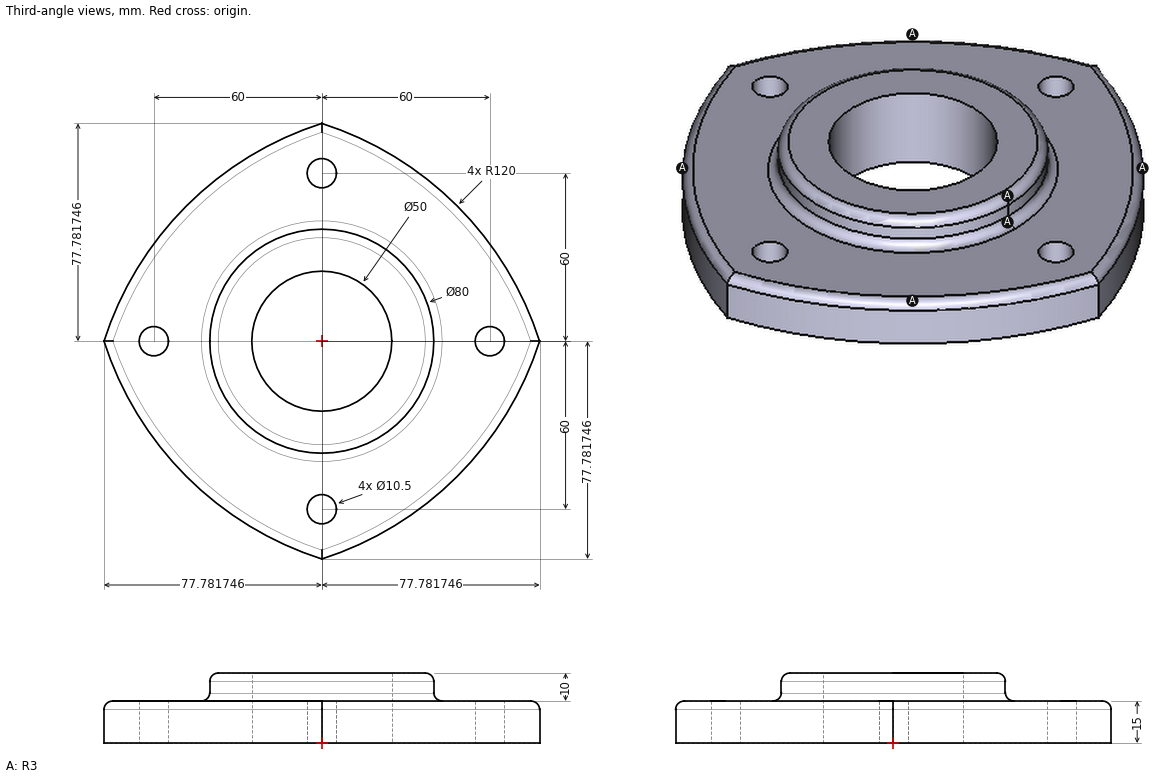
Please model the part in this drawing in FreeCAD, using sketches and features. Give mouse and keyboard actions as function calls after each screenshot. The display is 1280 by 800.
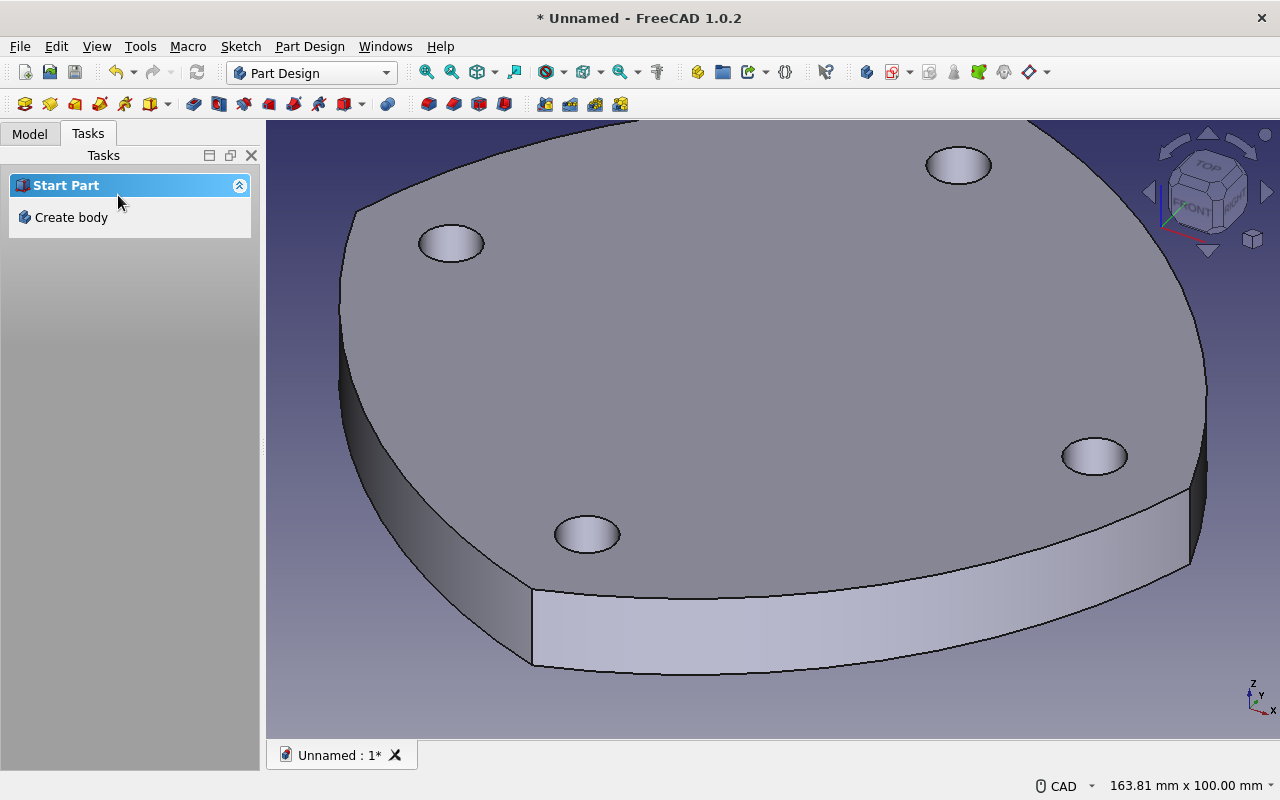
key(v)
key(f)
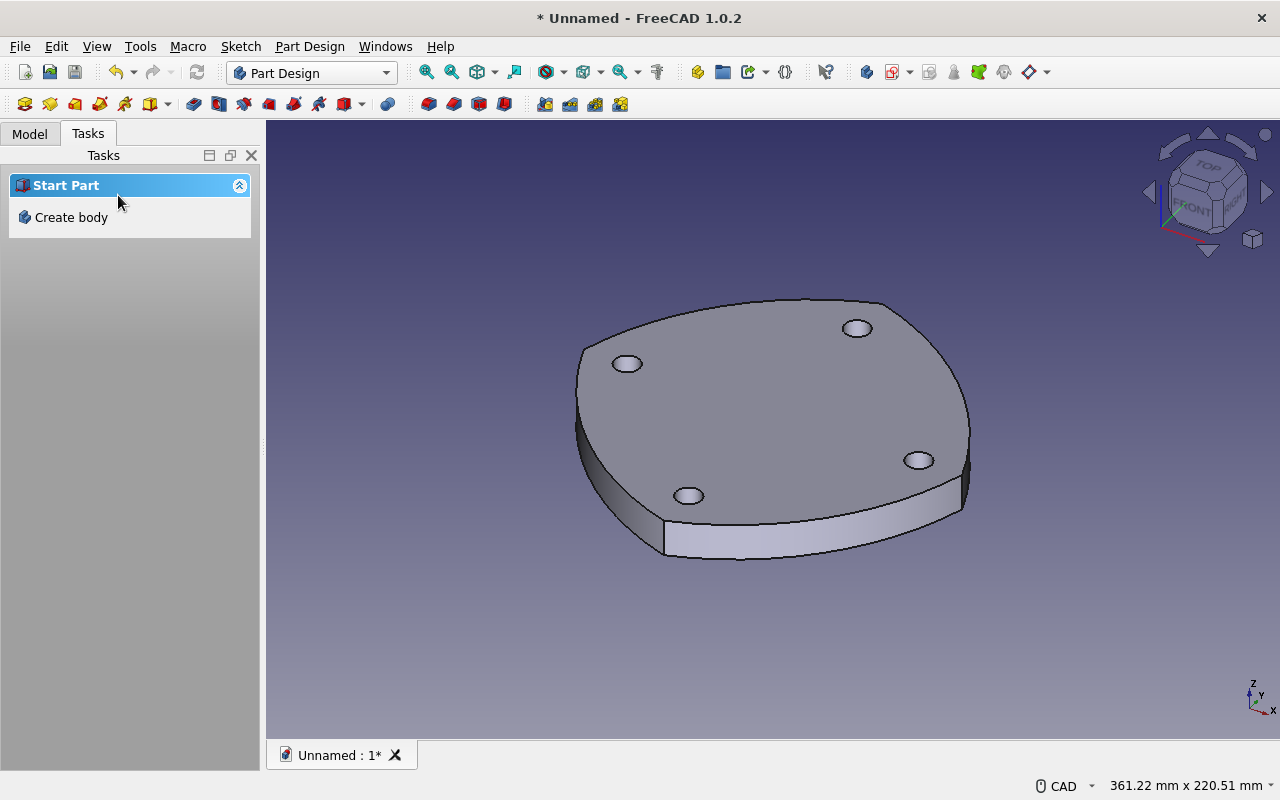
click(773, 411)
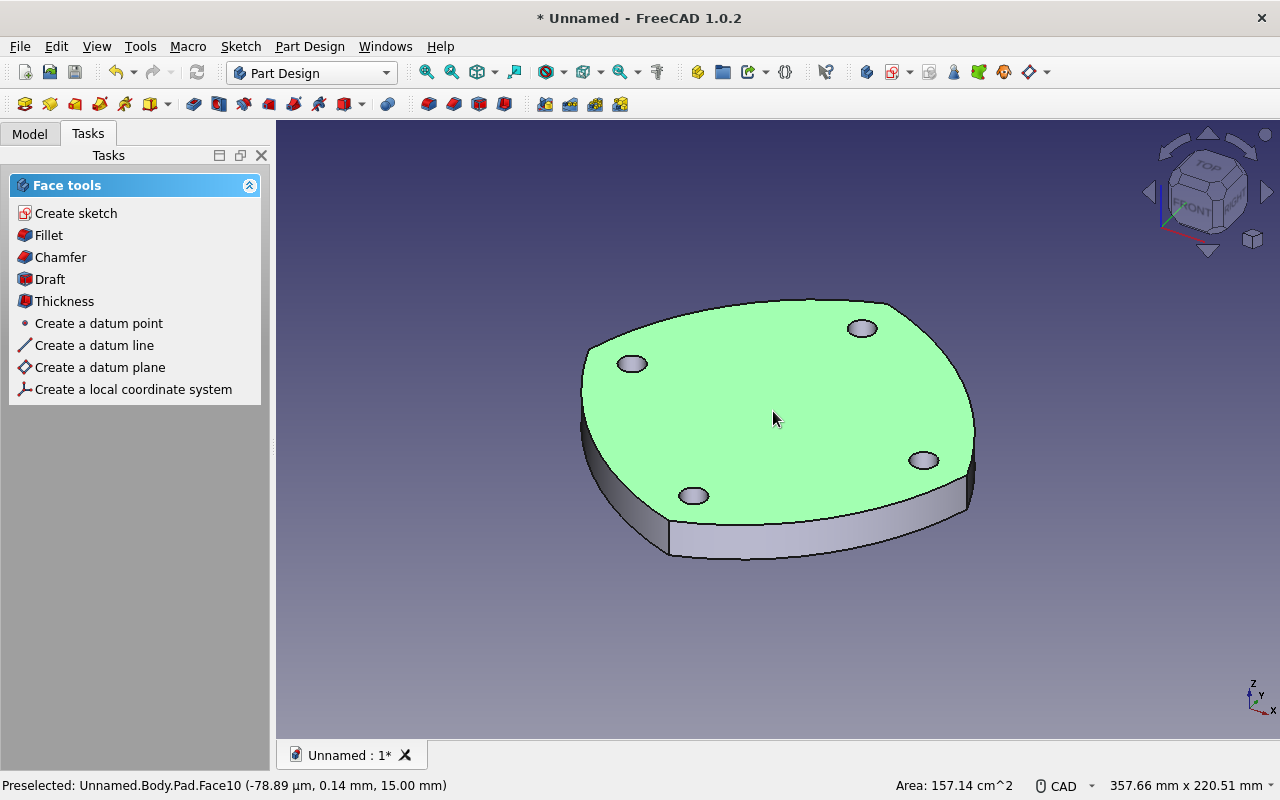
click(892, 72)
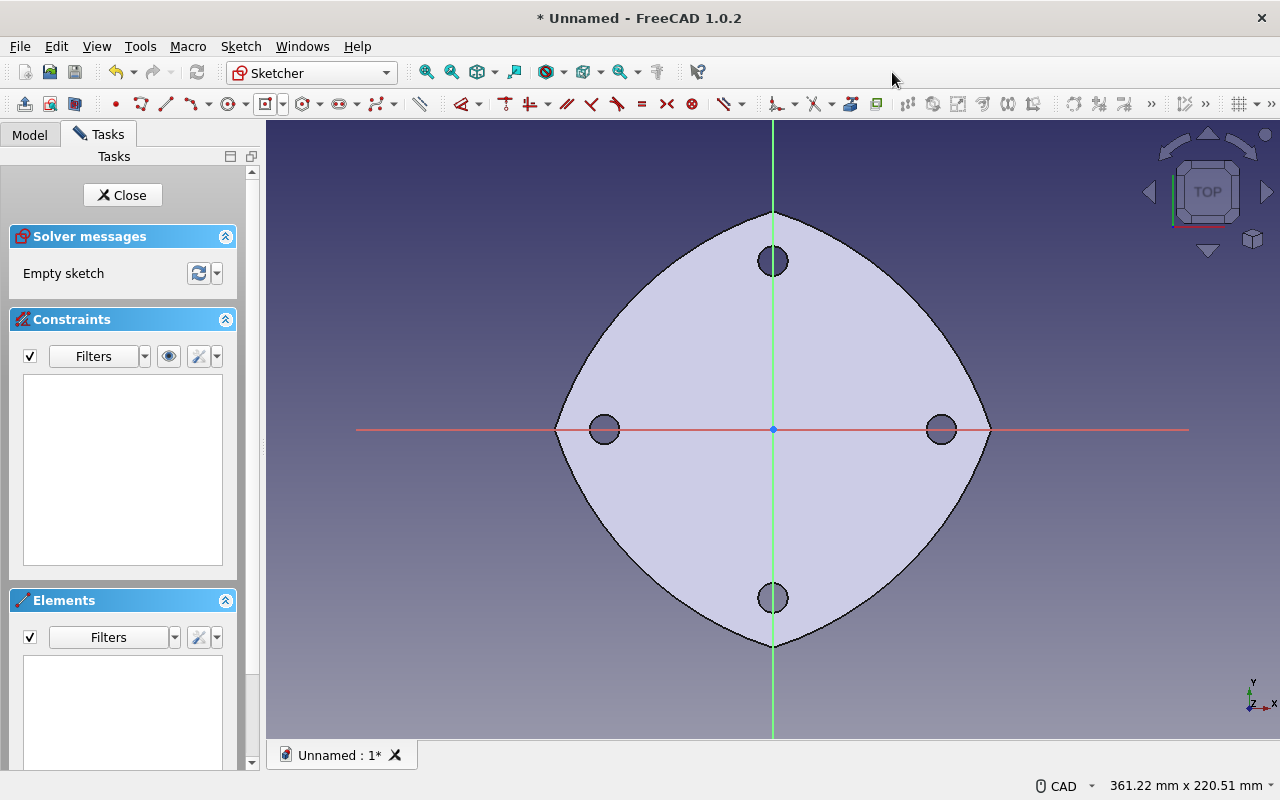
scroll(856, 430, up, 3)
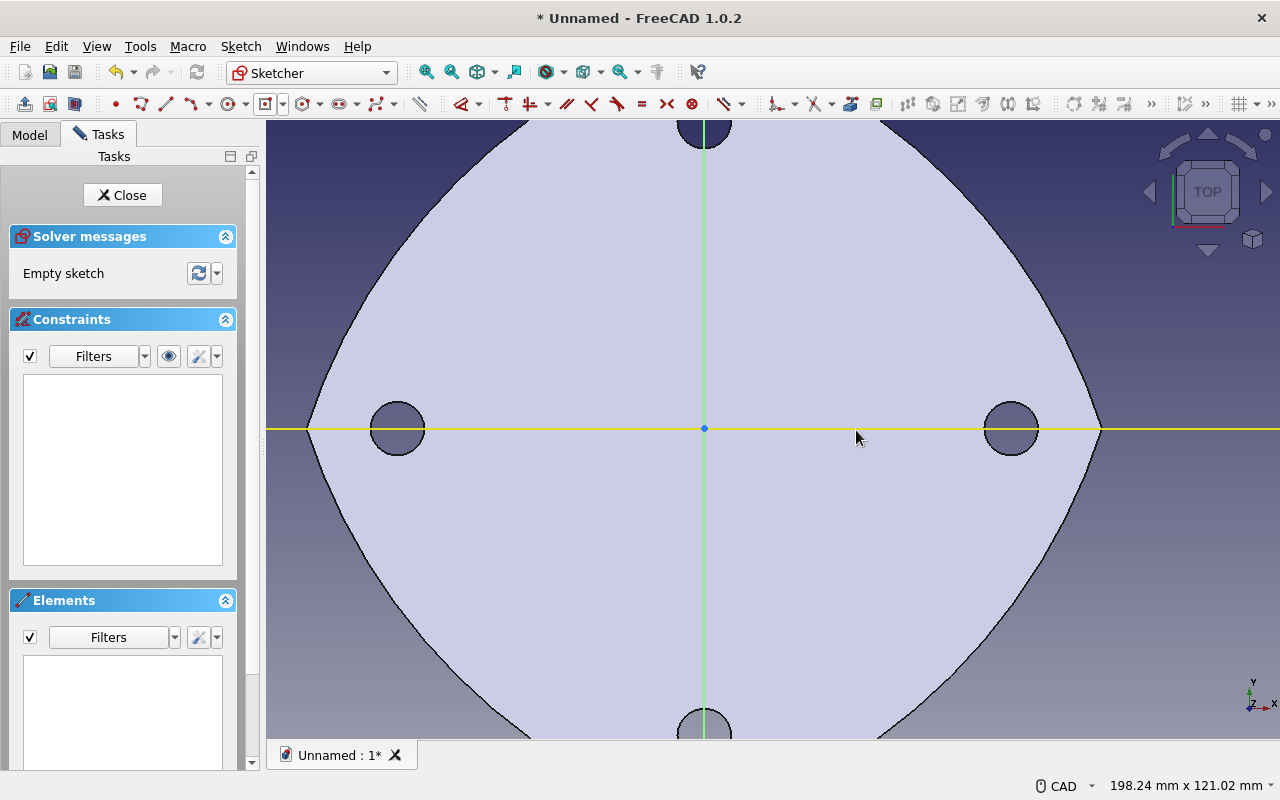
key(g)
key(c)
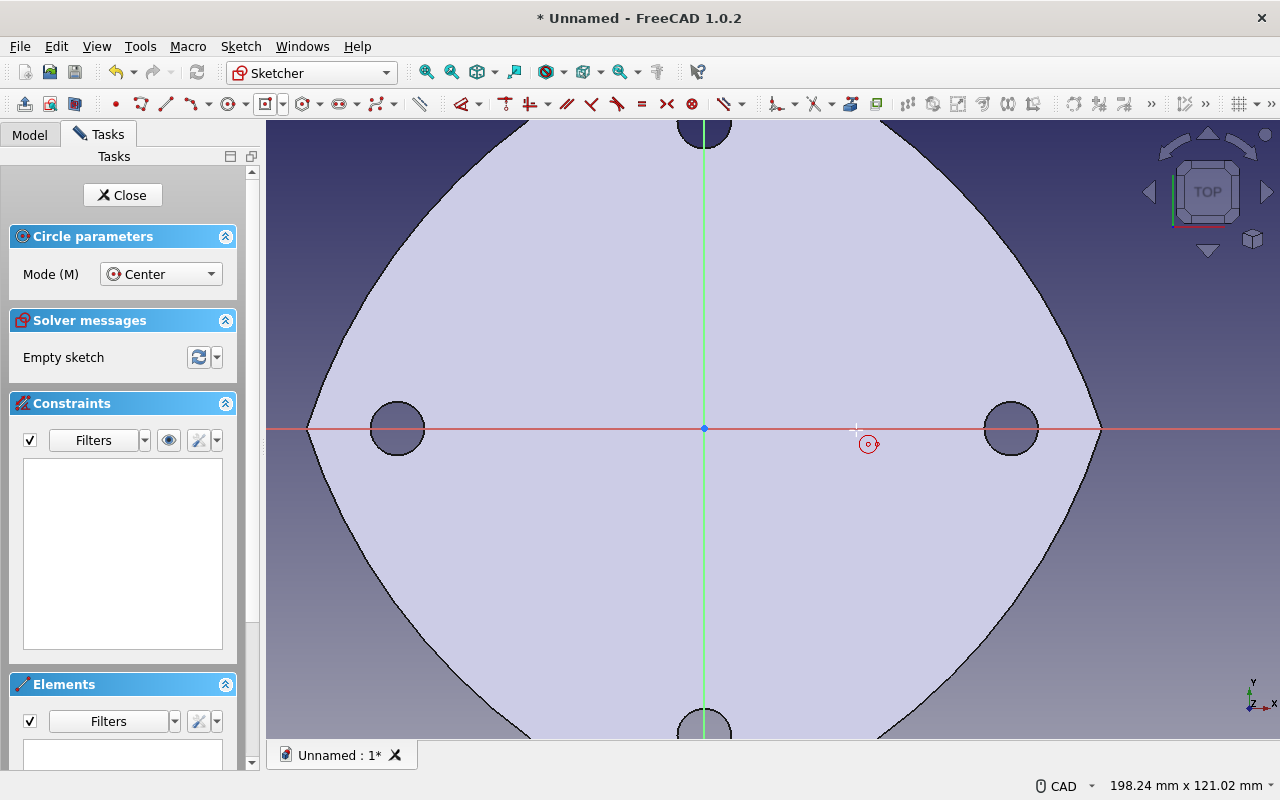
click(704, 429)
click(849, 284)
key(Escape)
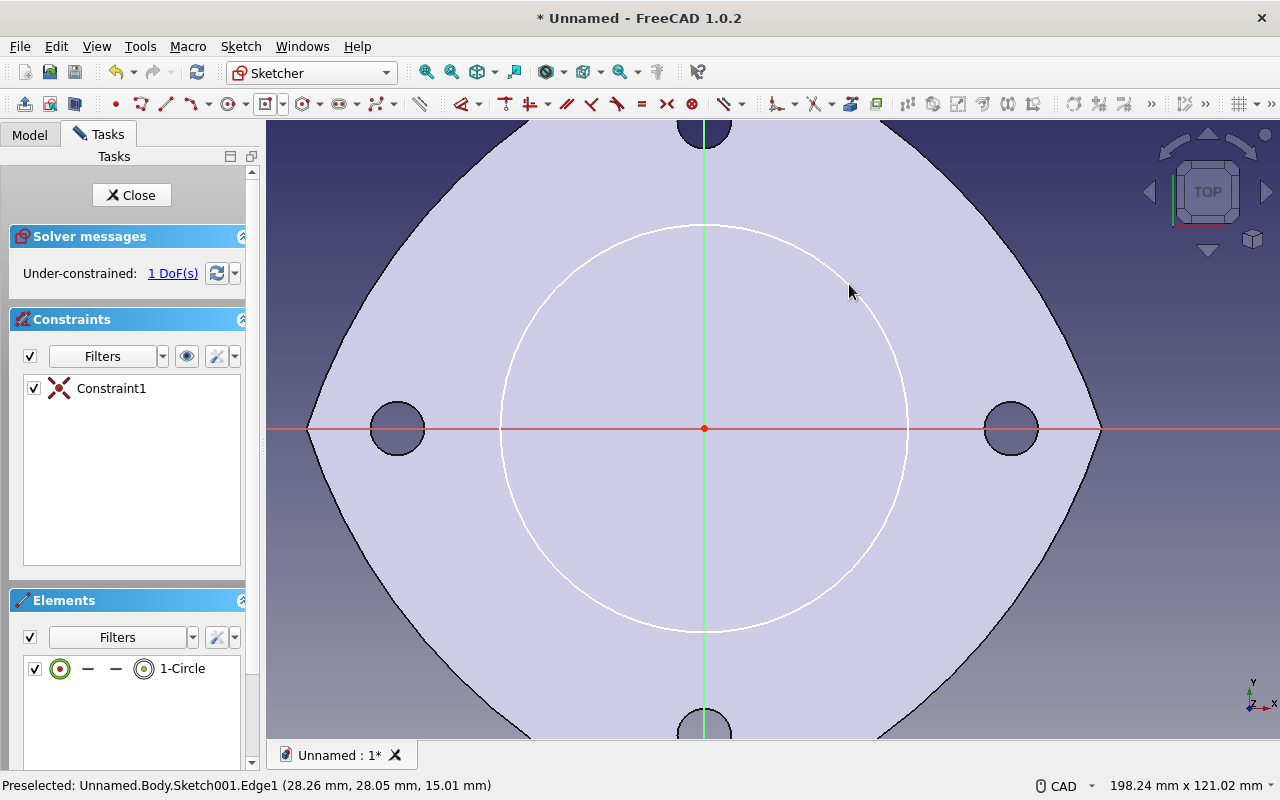
key(d)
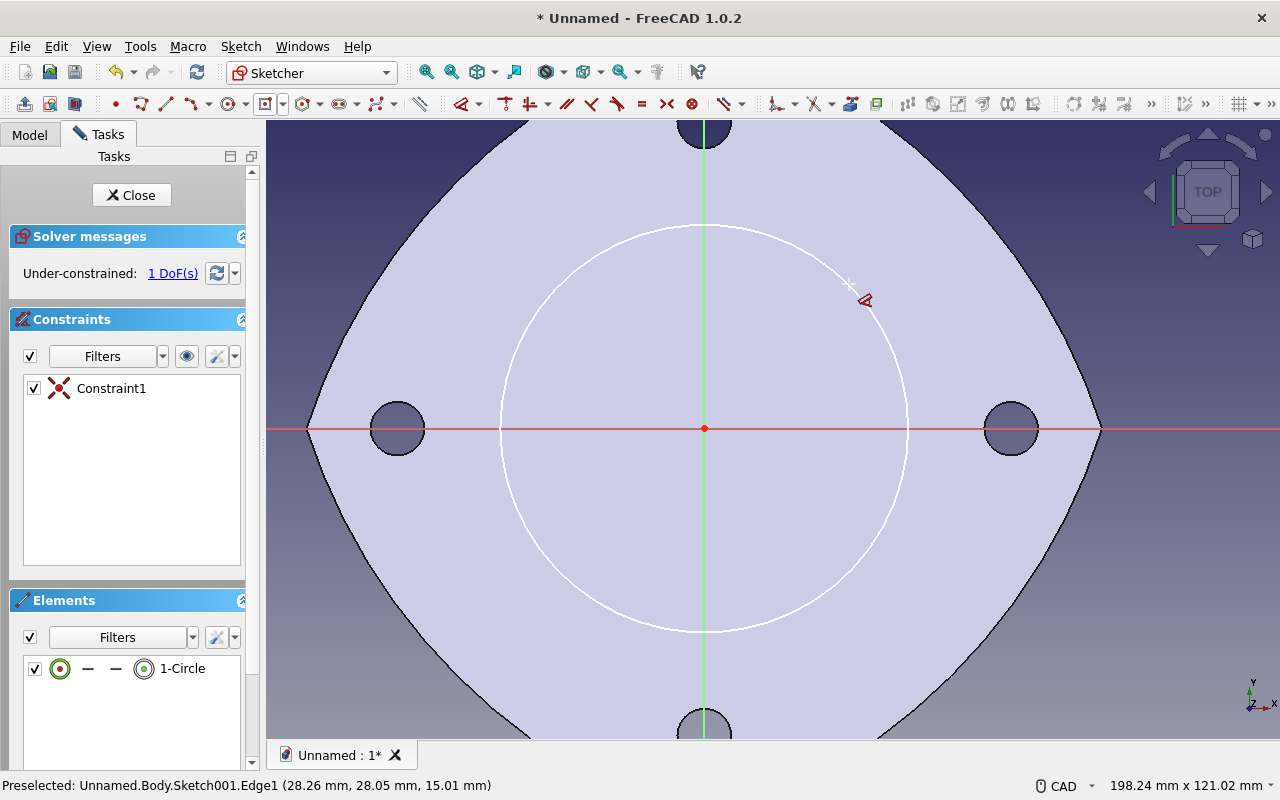
click(848, 284)
click(871, 261)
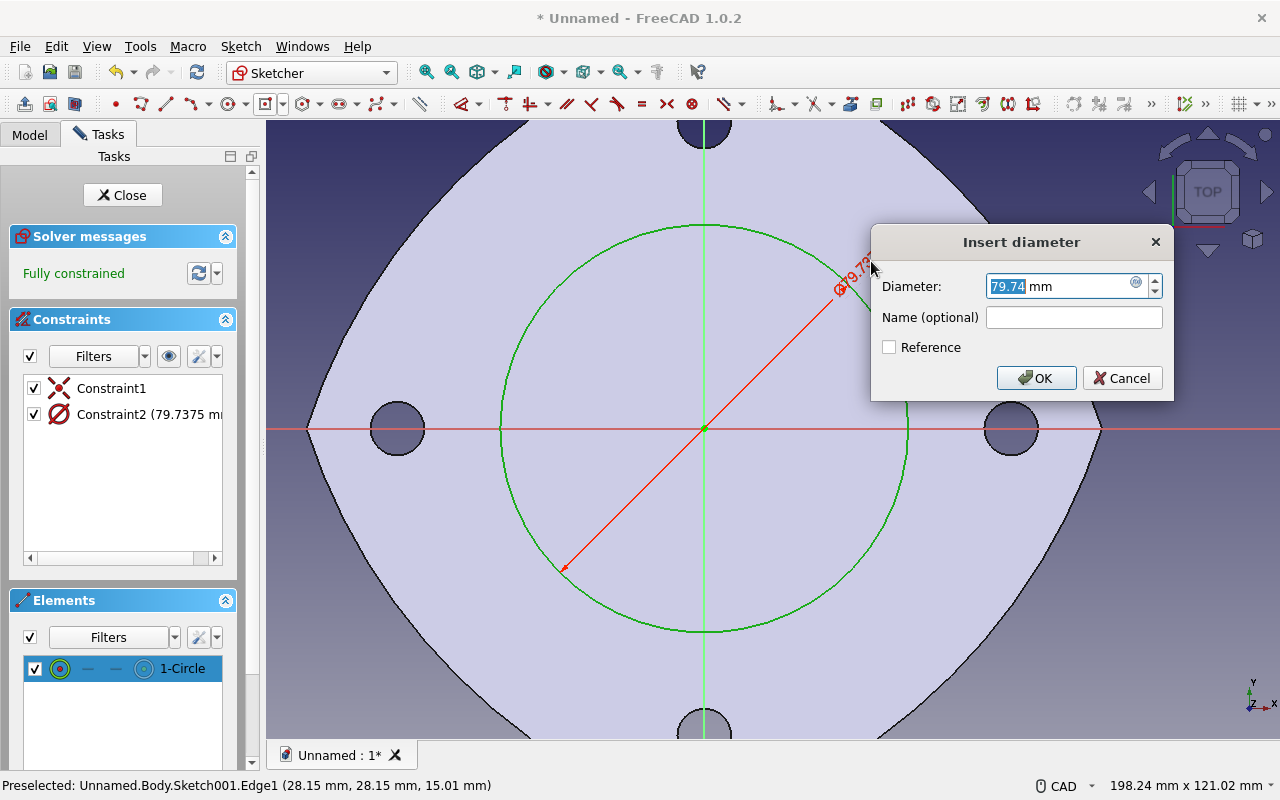
text(80)
key(Return)
key(Escape)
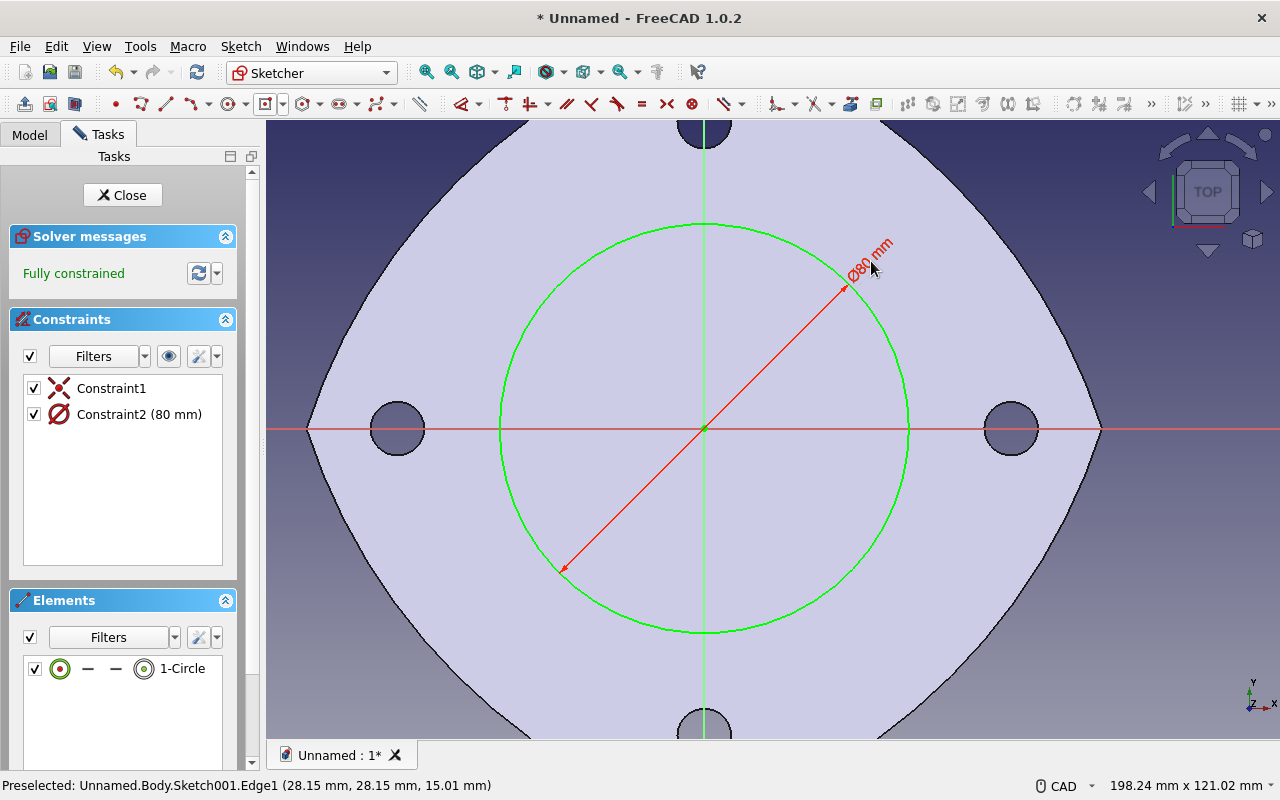
click(123, 195)